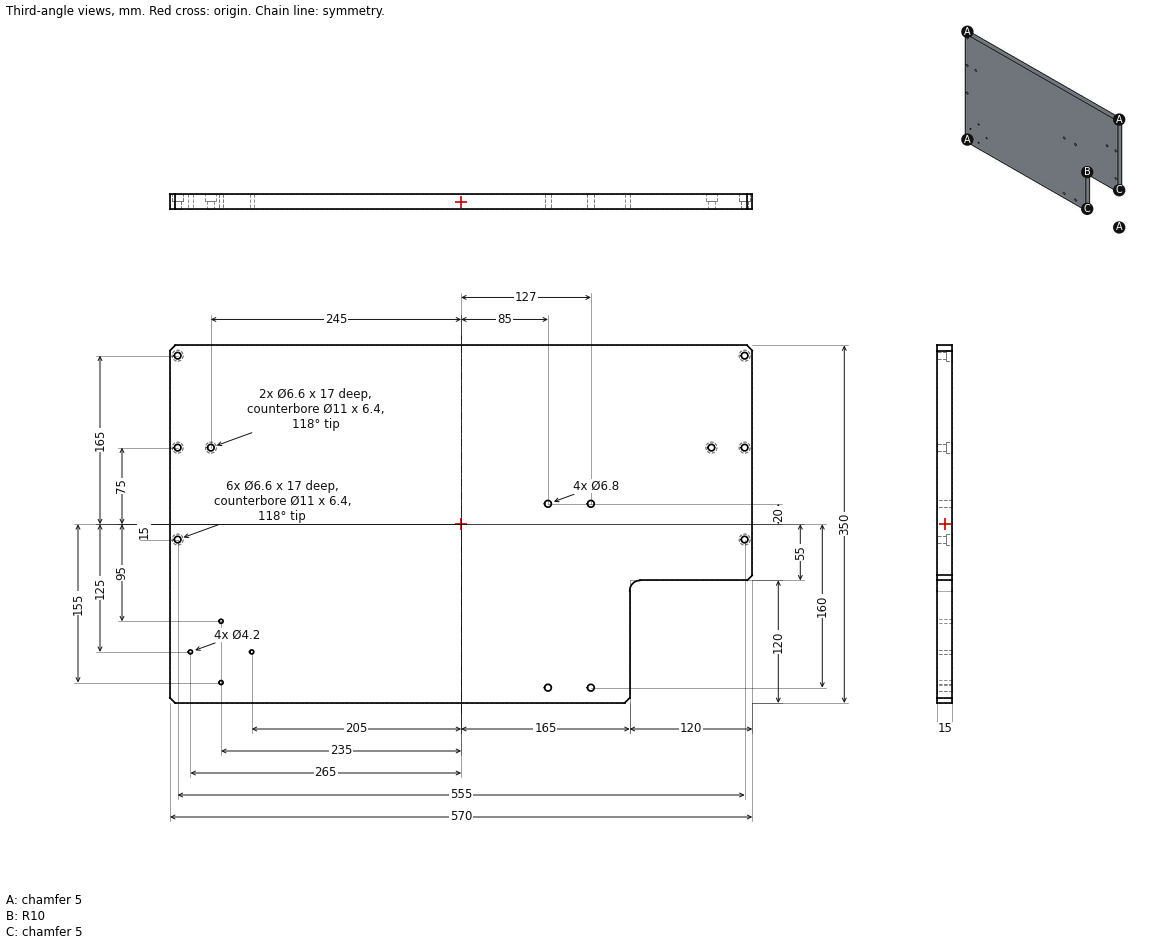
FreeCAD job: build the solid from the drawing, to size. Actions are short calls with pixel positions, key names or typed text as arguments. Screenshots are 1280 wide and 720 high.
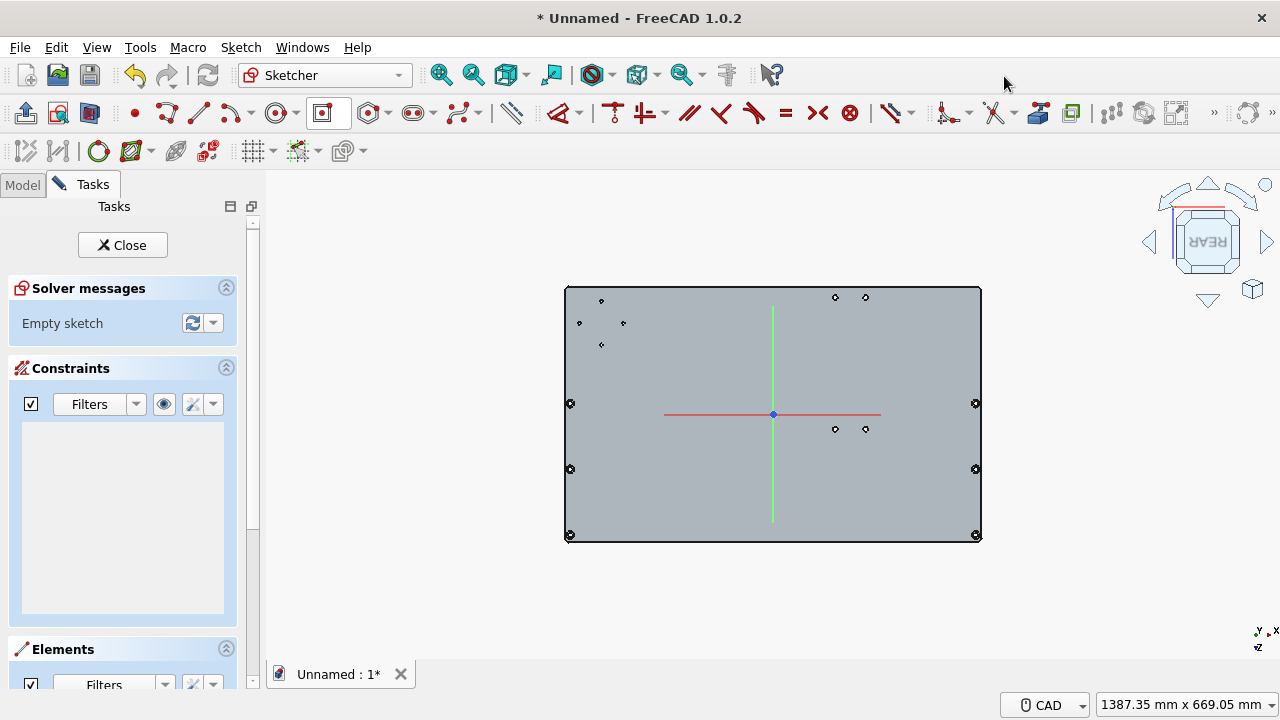
scroll(912, 501, up, 2)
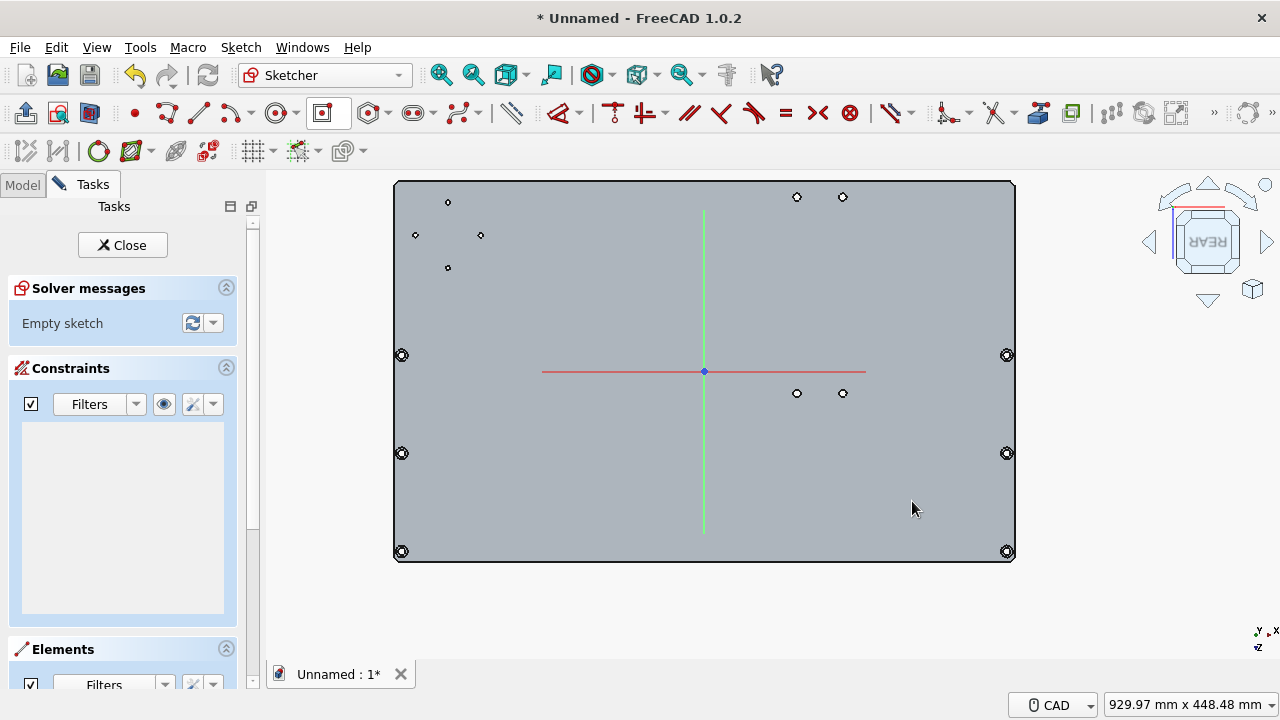
click(276, 114)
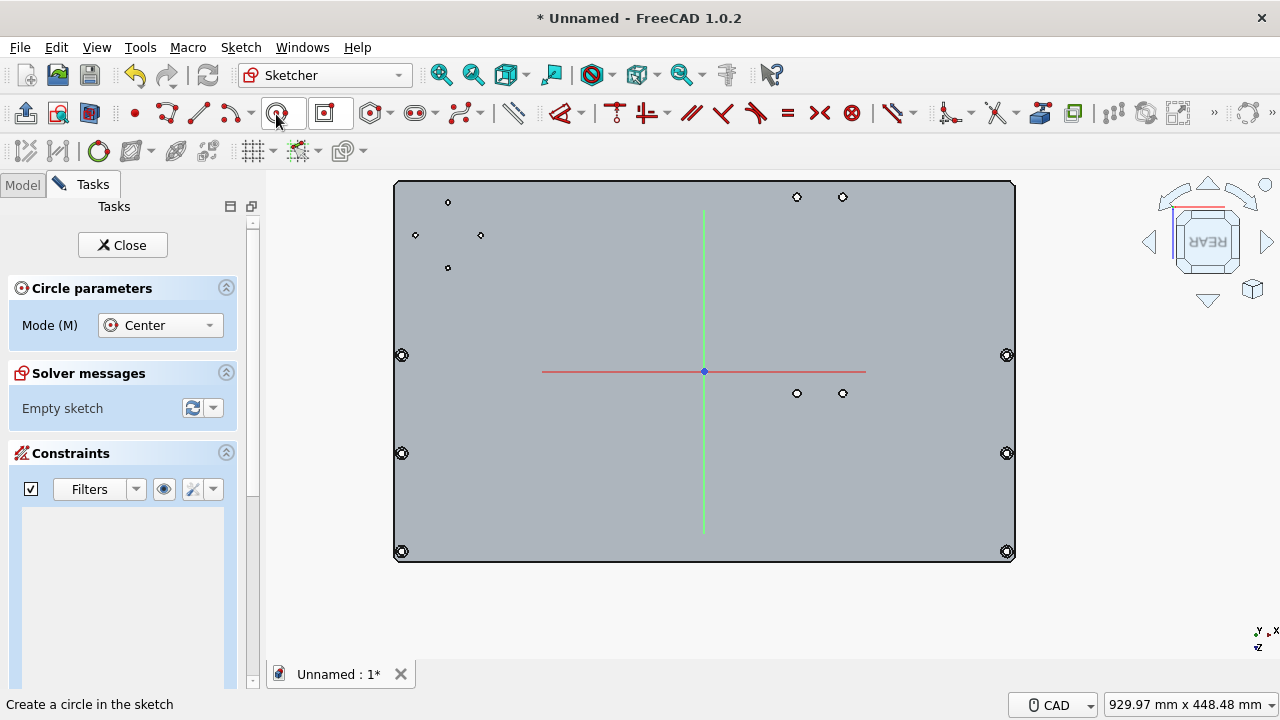
scroll(437, 453, up, 10)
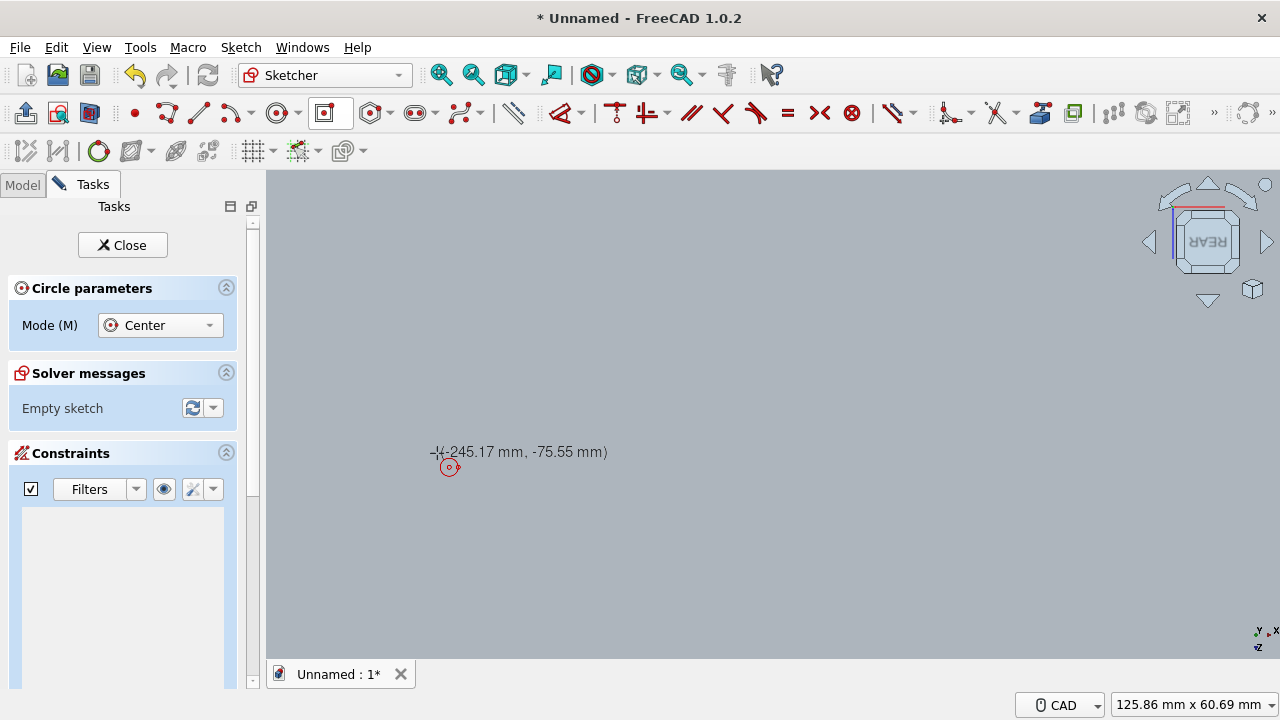
scroll(437, 454, down, 10)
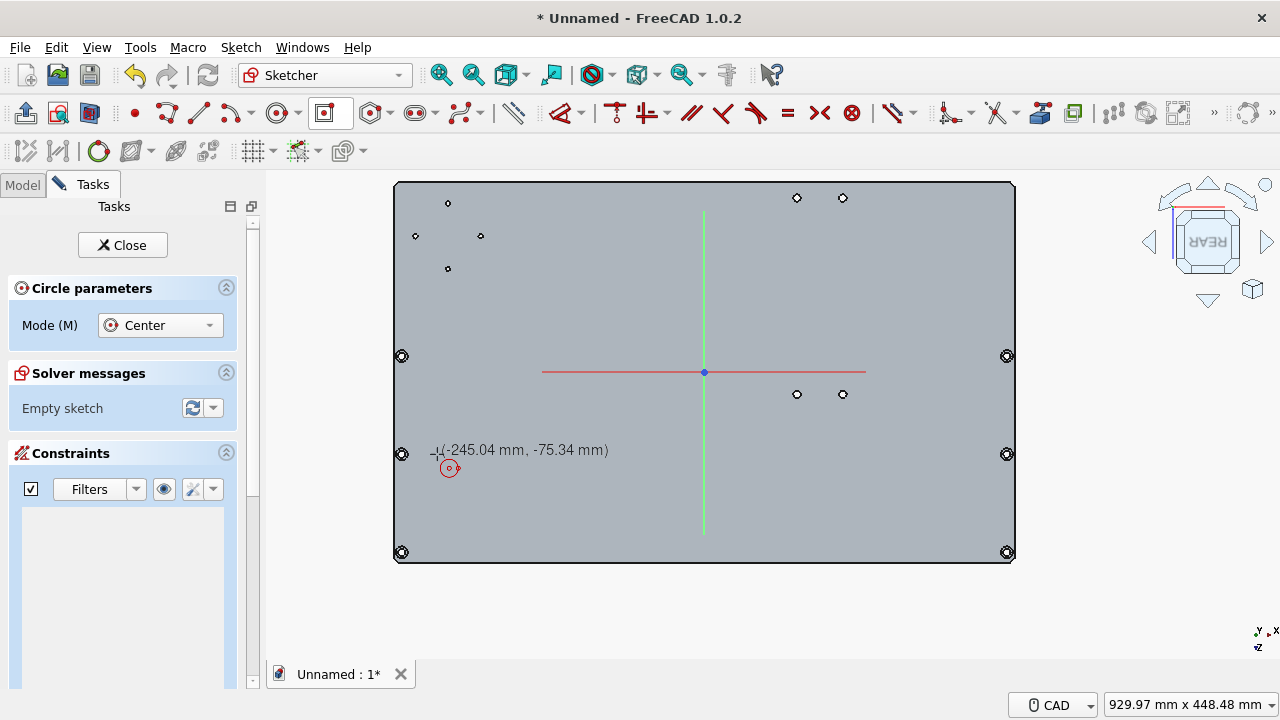
click(437, 454)
move(440, 452)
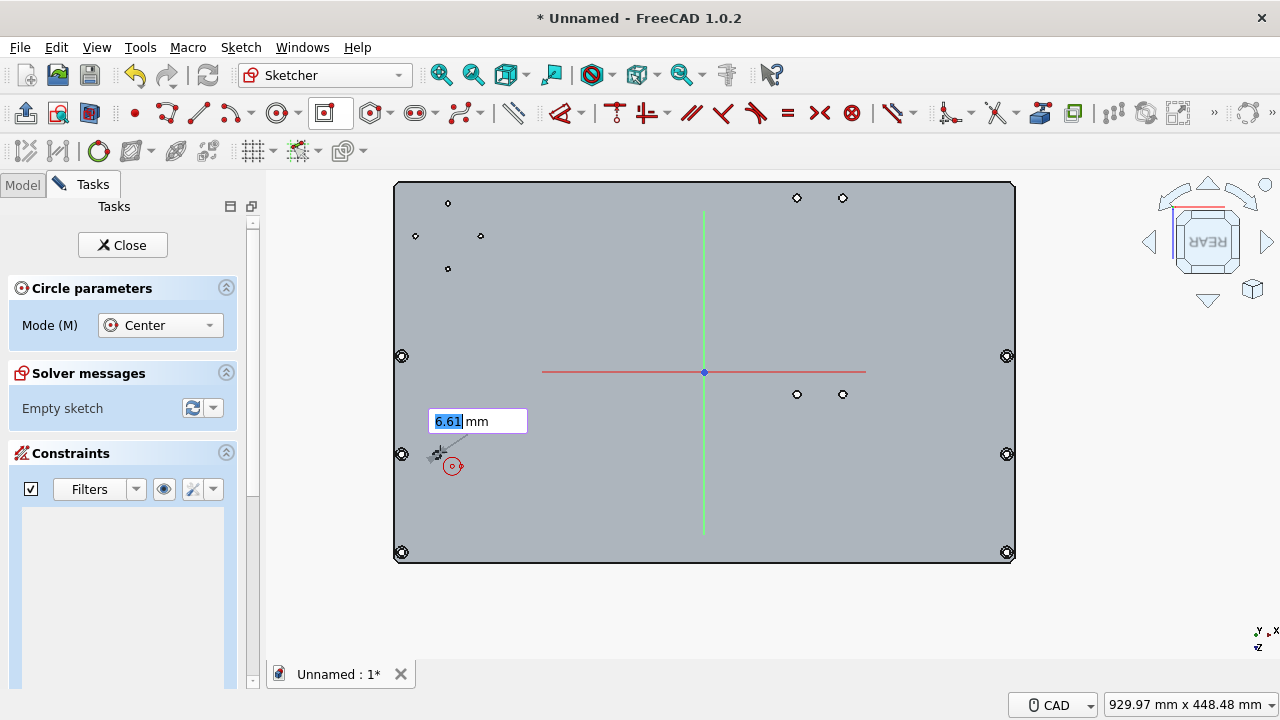
text(6.6)
key(Return)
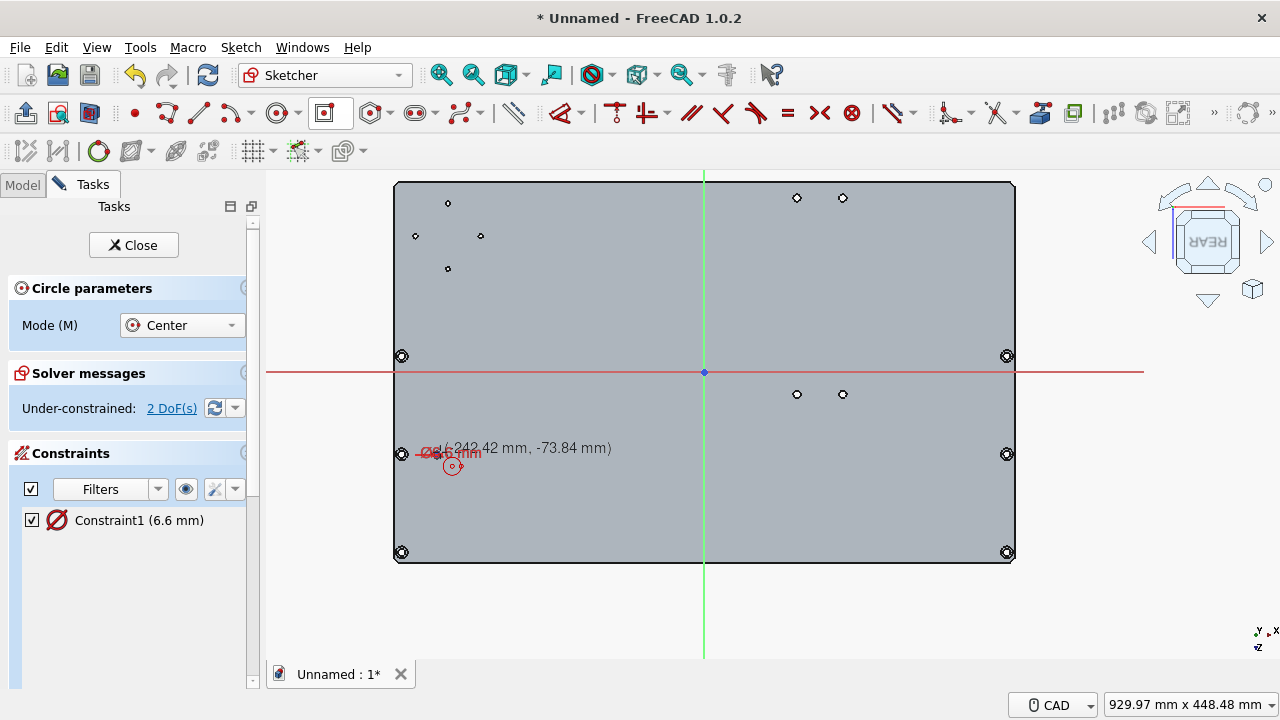
scroll(971, 454, up, 10)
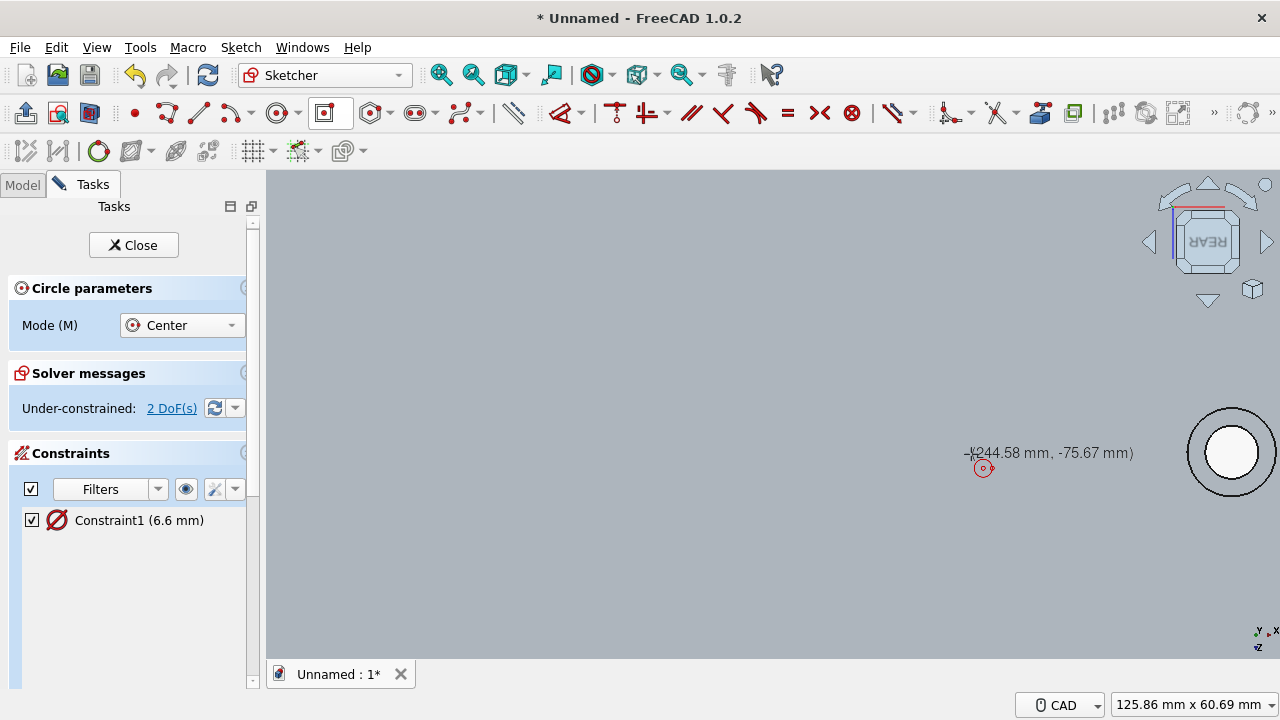
scroll(972, 454, down, 10)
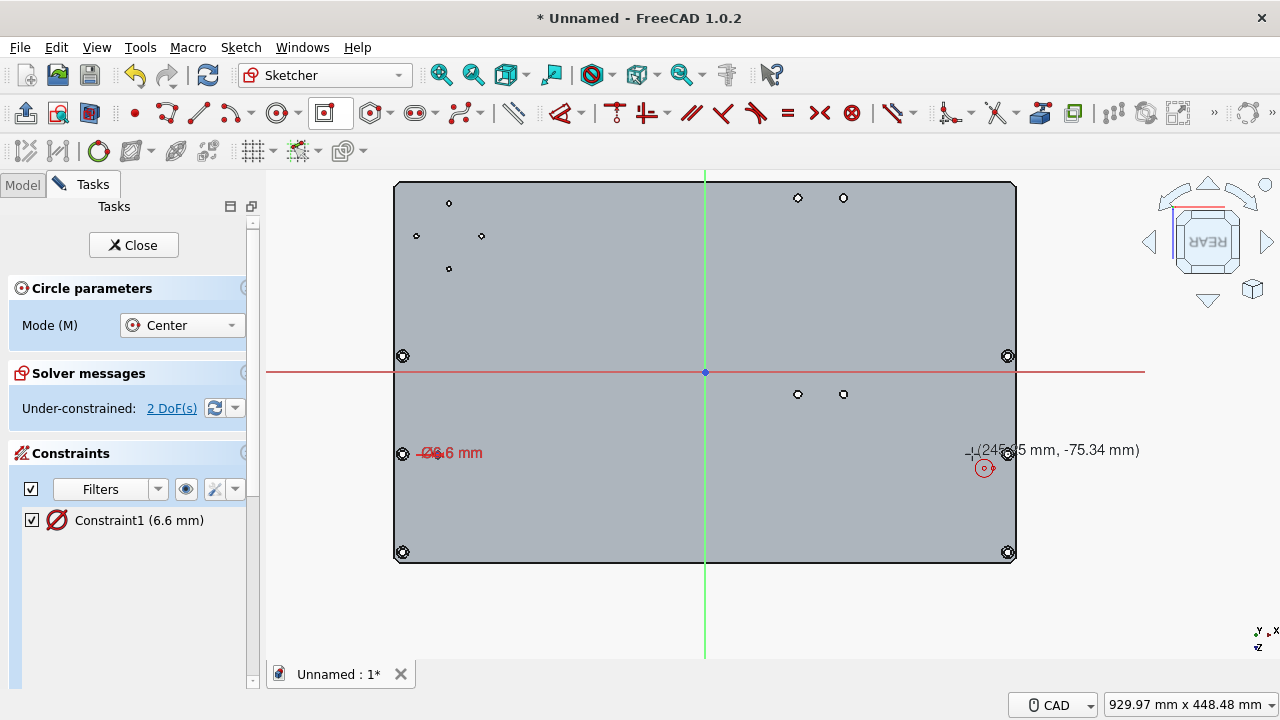
click(972, 454)
move(975, 452)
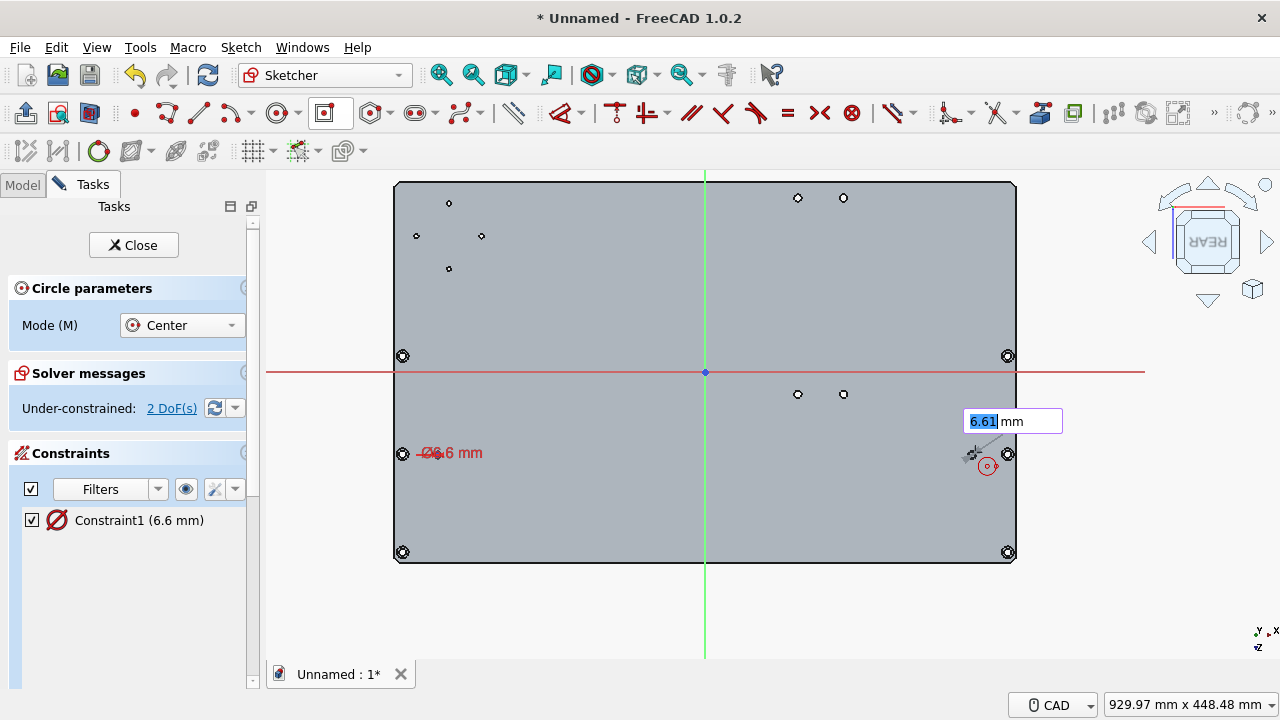
text(6.6)
key(Return)
key(Escape)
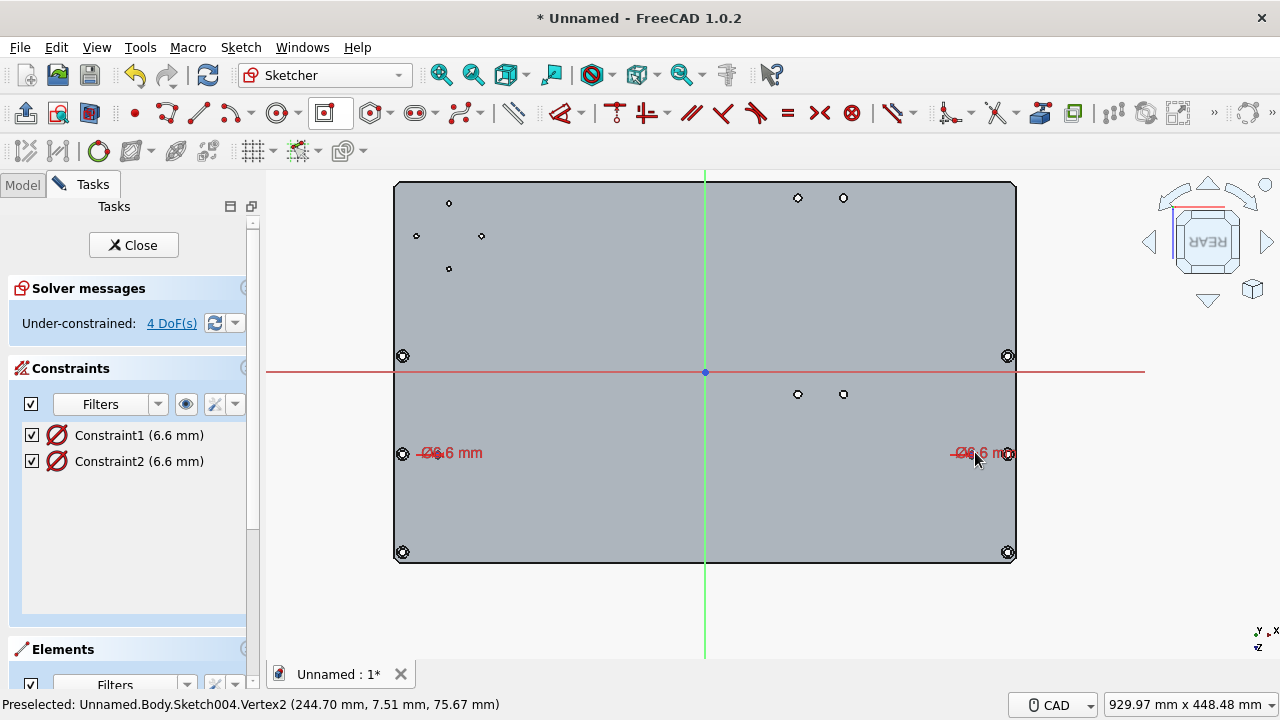
click(438, 455)